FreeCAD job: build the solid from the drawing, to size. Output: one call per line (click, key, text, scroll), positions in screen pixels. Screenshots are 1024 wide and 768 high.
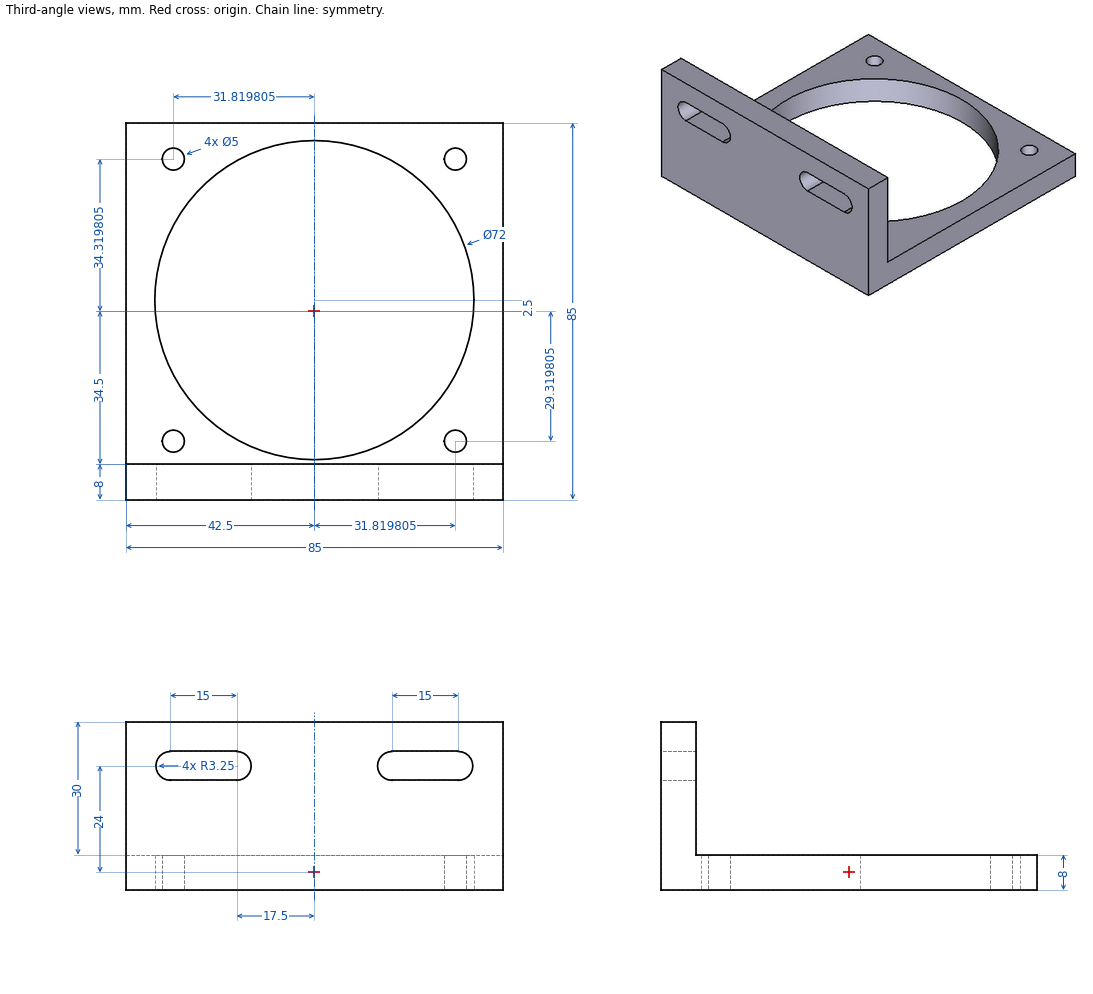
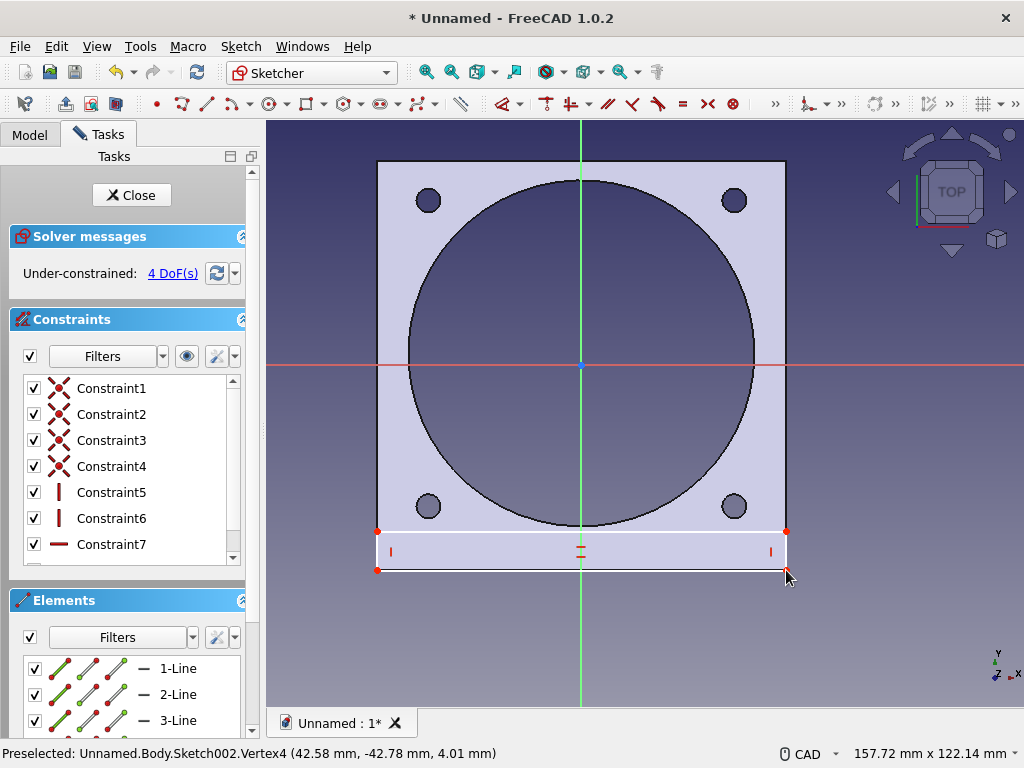
key(d)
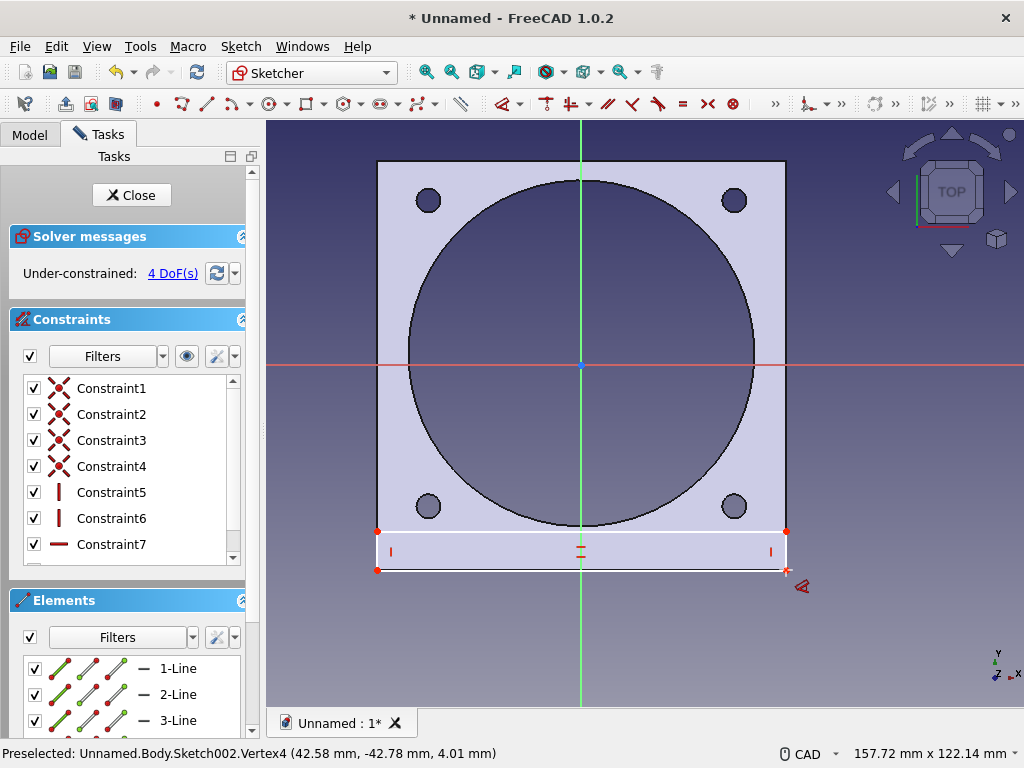
click(377, 544)
click(343, 551)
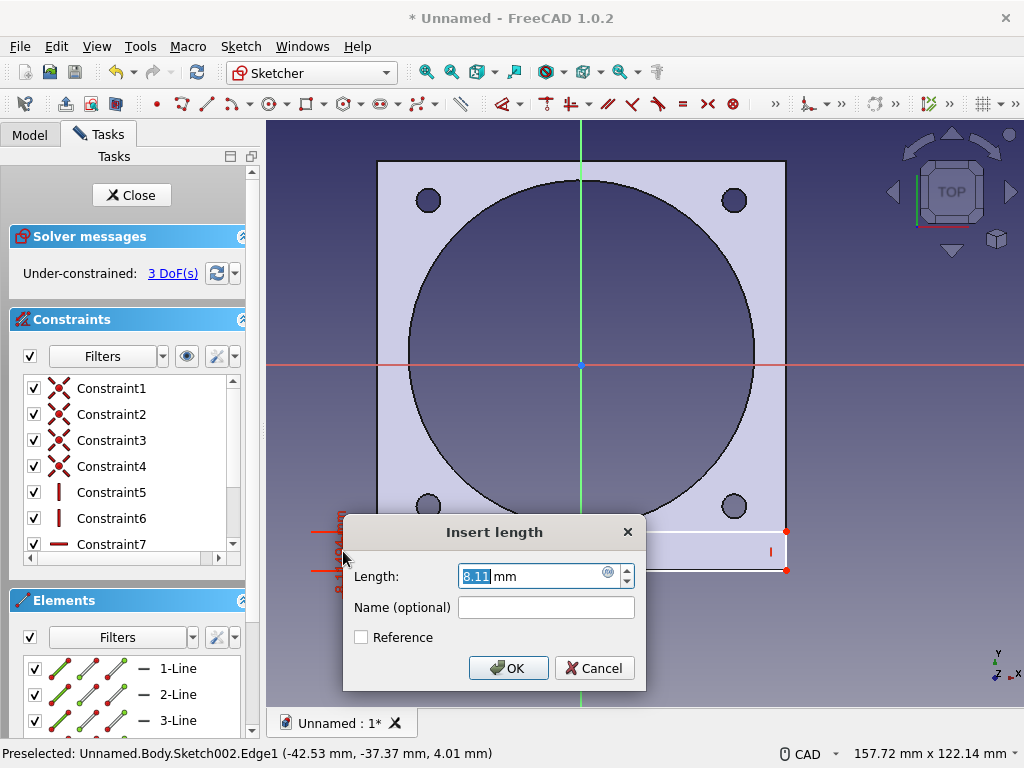
text(8)
key(Return)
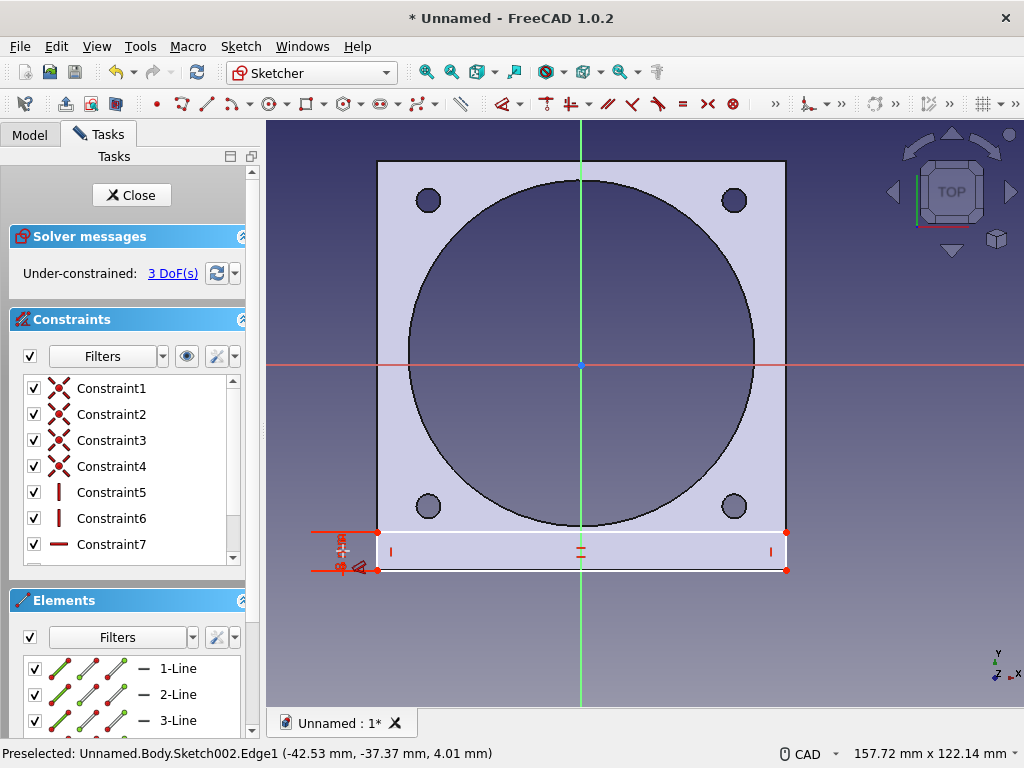
click(500, 571)
click(487, 605)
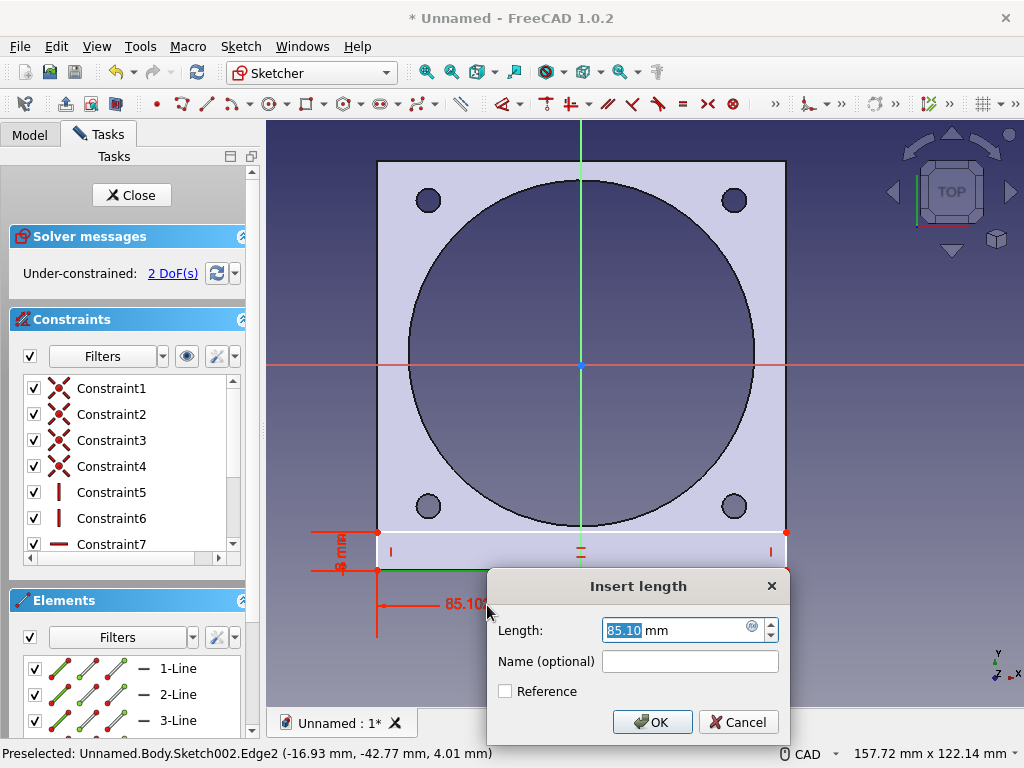
text(85)
key(Return)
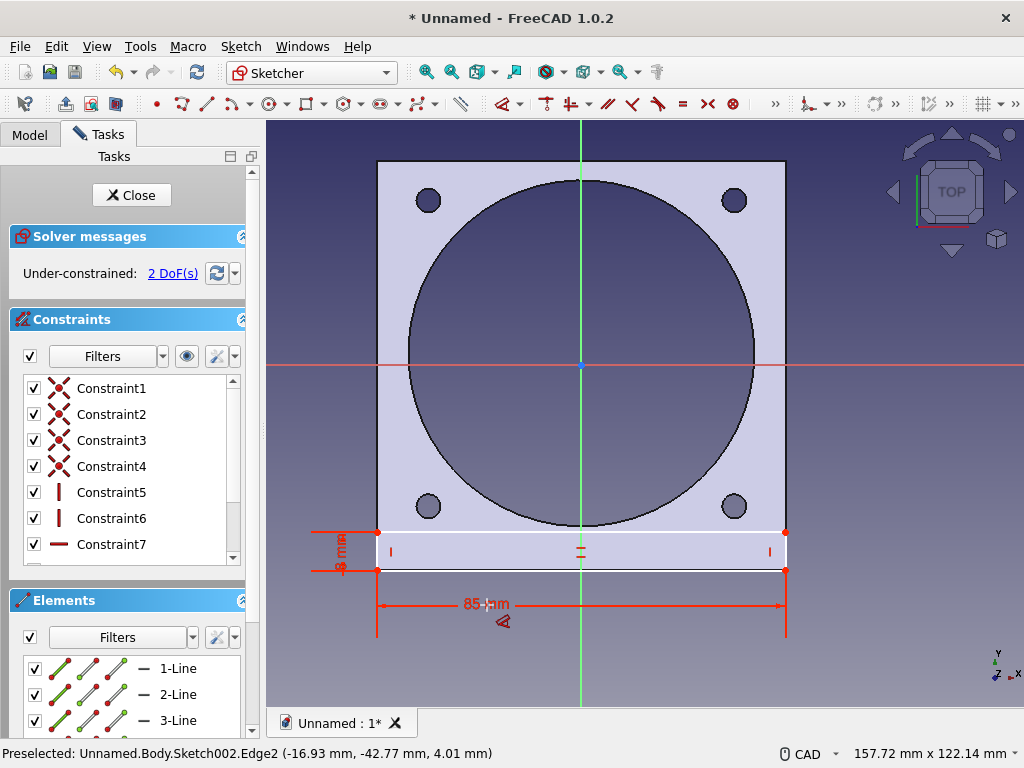
click(377, 532)
click(479, 331)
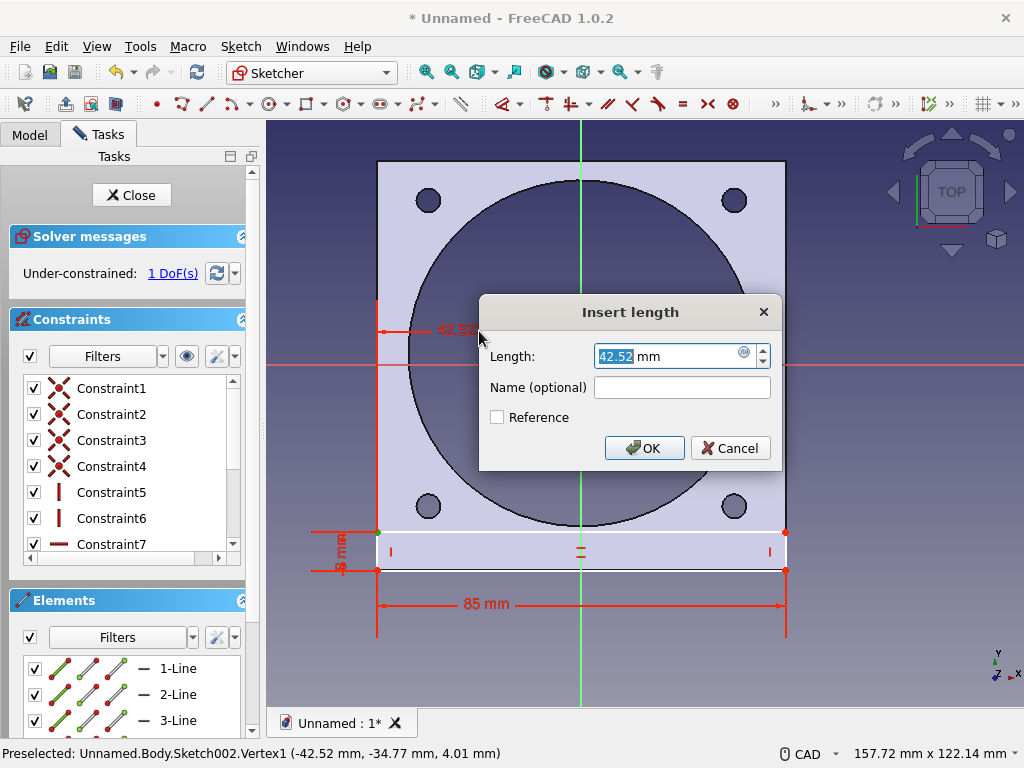
text(42.5)
key(Return)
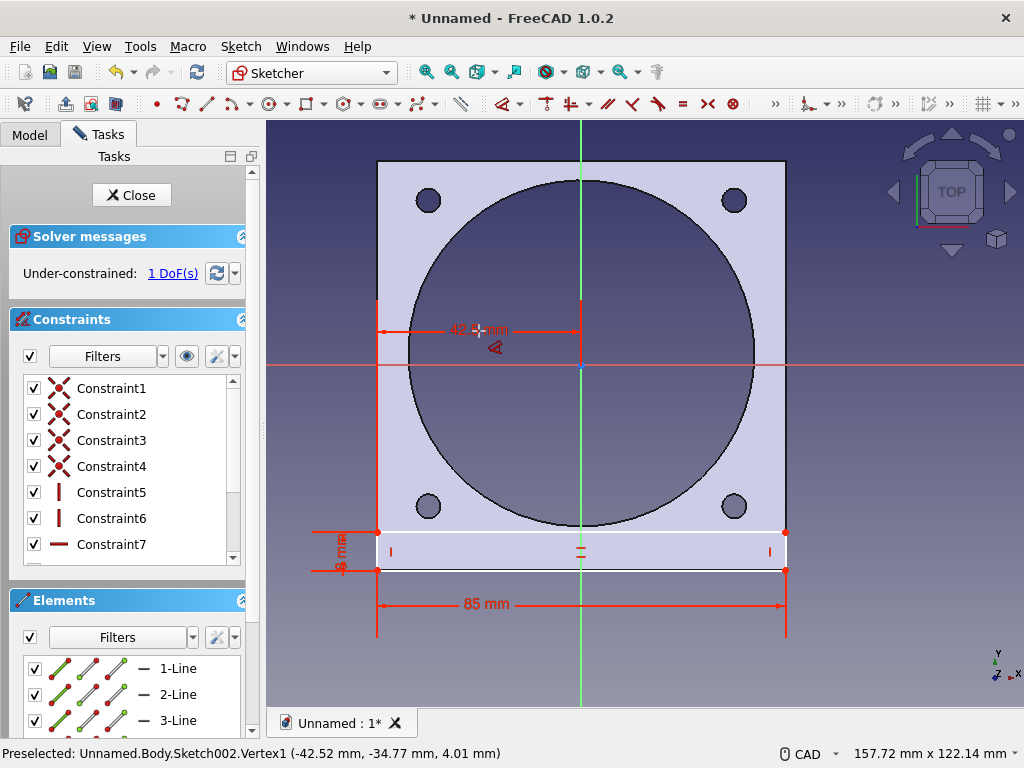
click(377, 532)
click(343, 449)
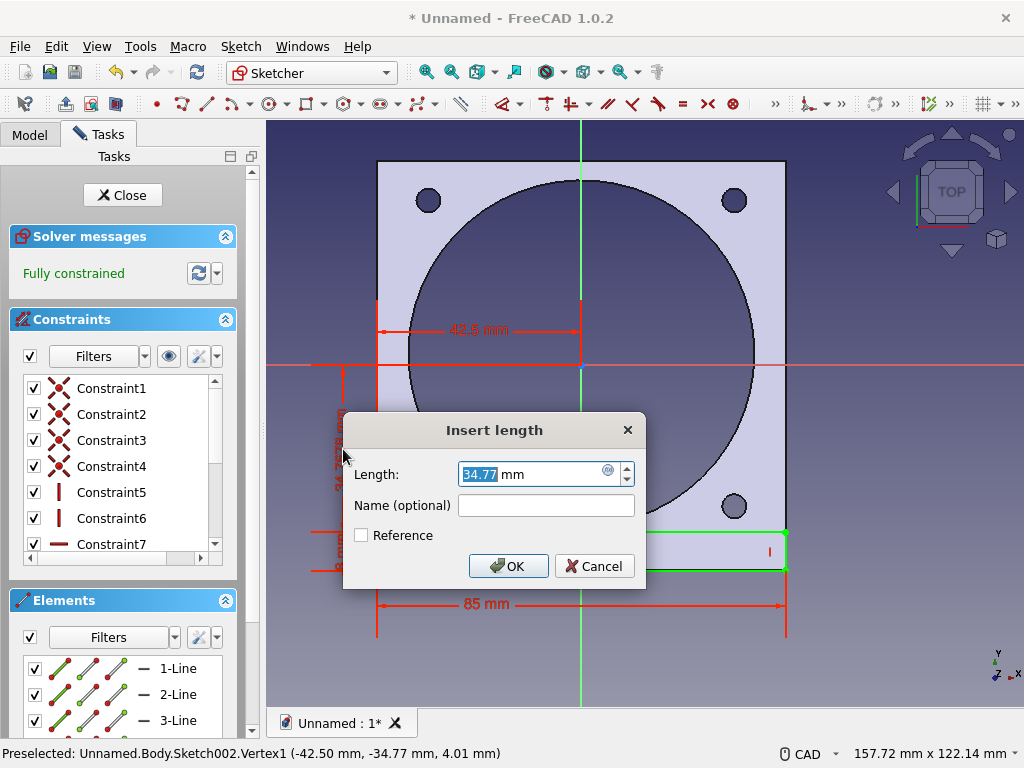
text(34.5)
key(Return)
key(Escape)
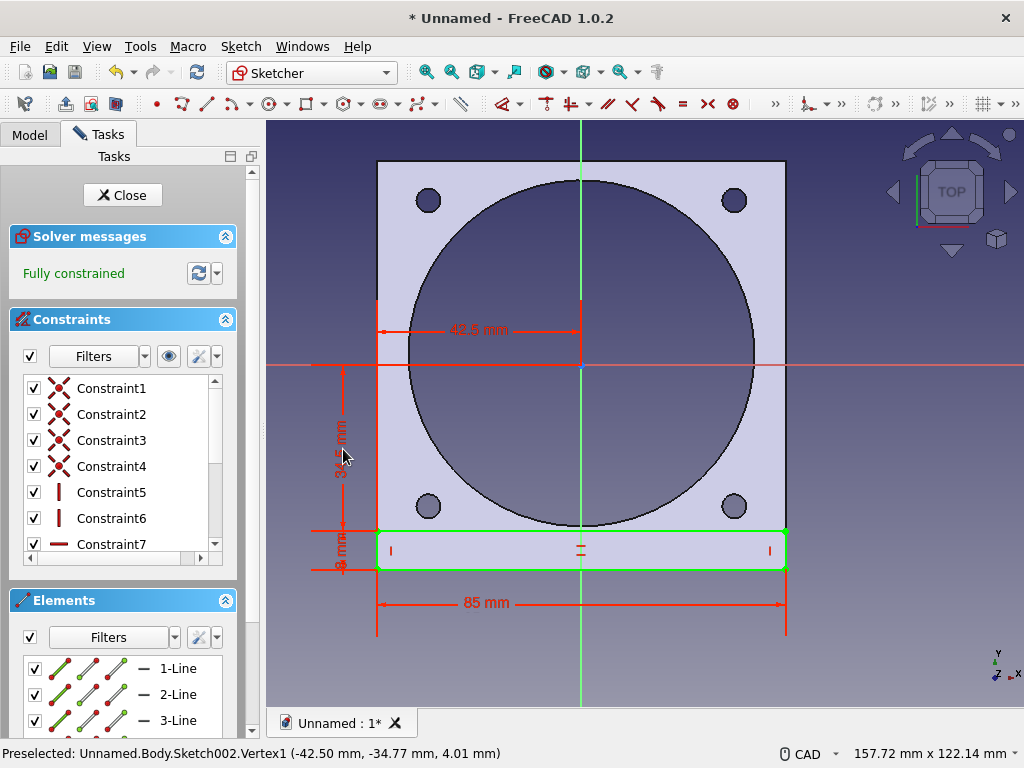
click(123, 195)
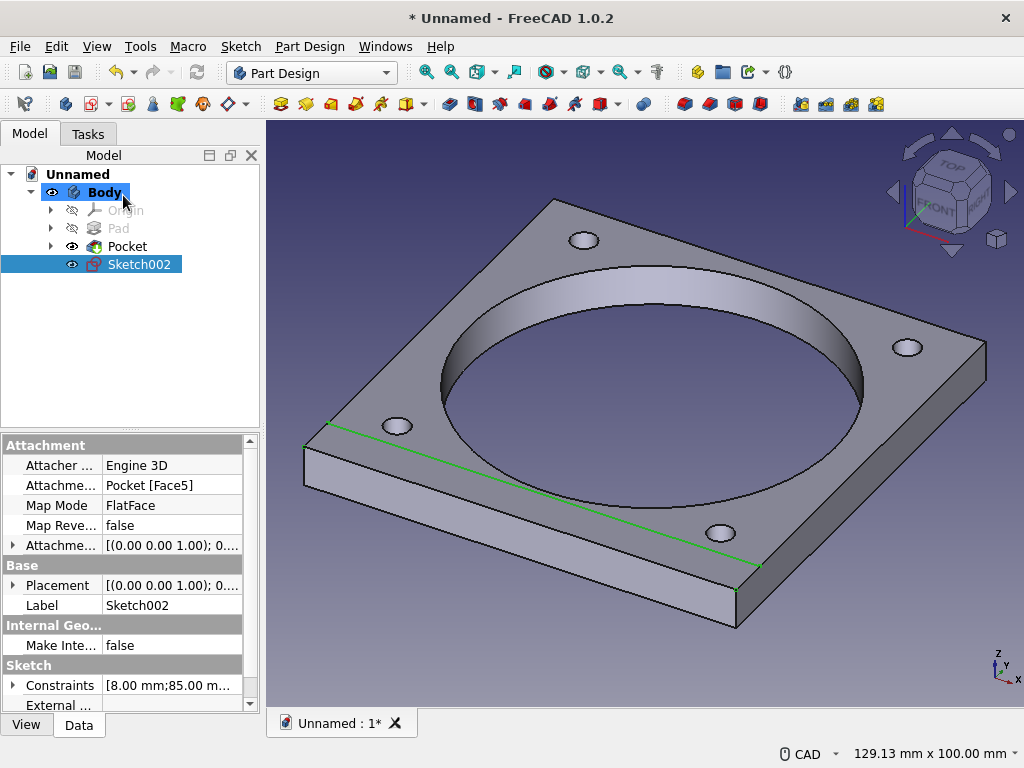
click(281, 104)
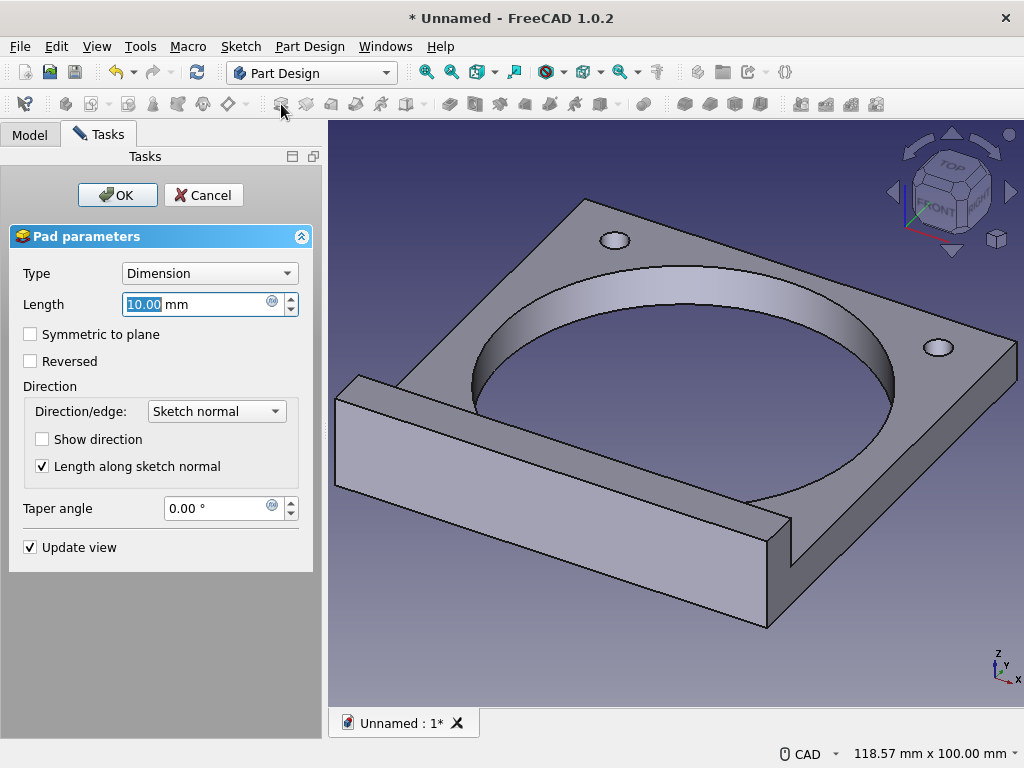
text(30)
key(Tab)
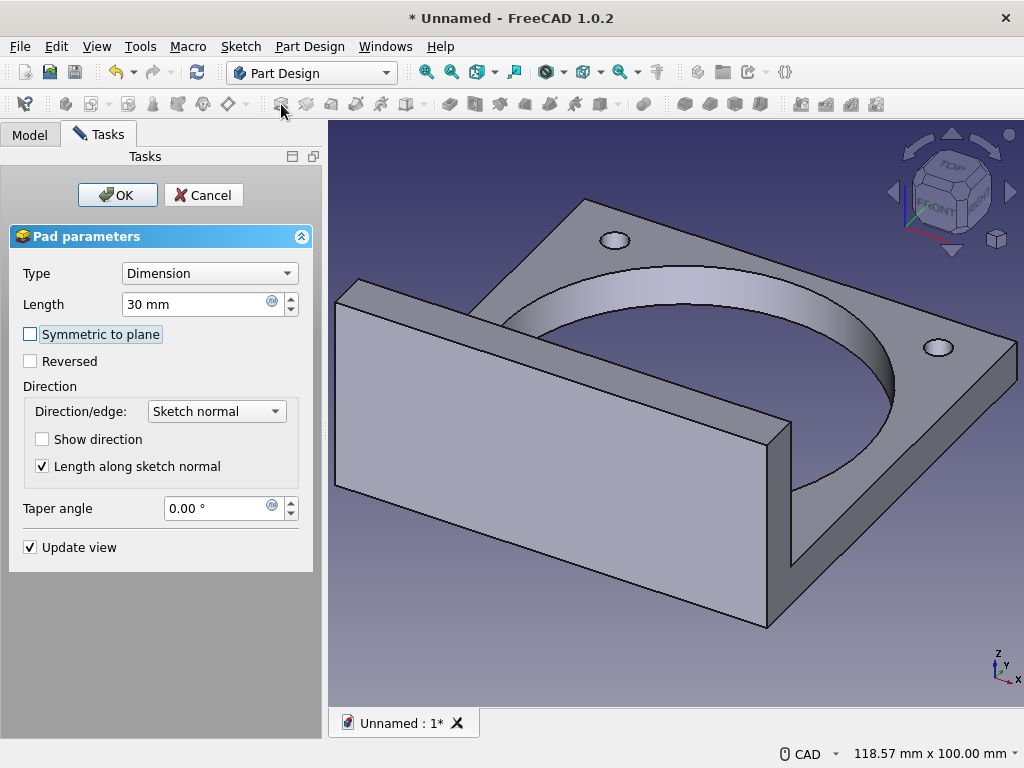
click(118, 195)